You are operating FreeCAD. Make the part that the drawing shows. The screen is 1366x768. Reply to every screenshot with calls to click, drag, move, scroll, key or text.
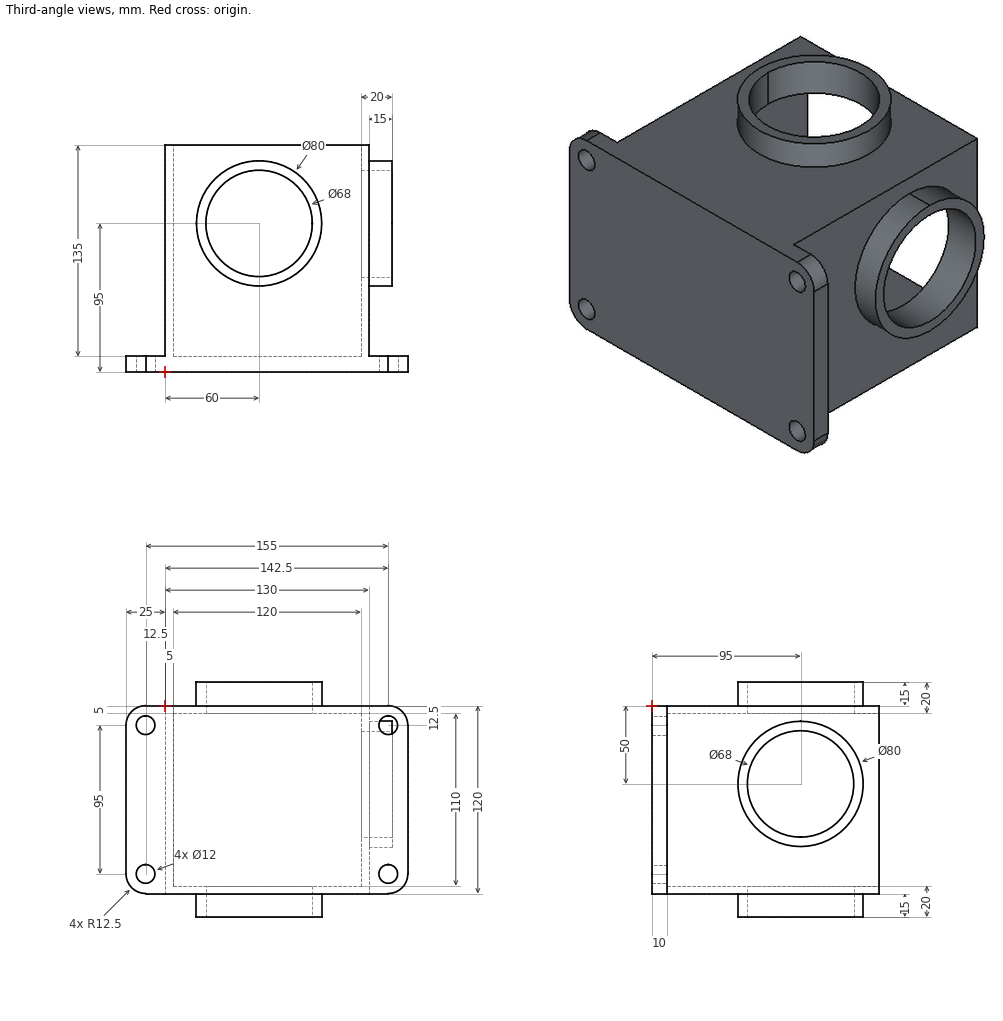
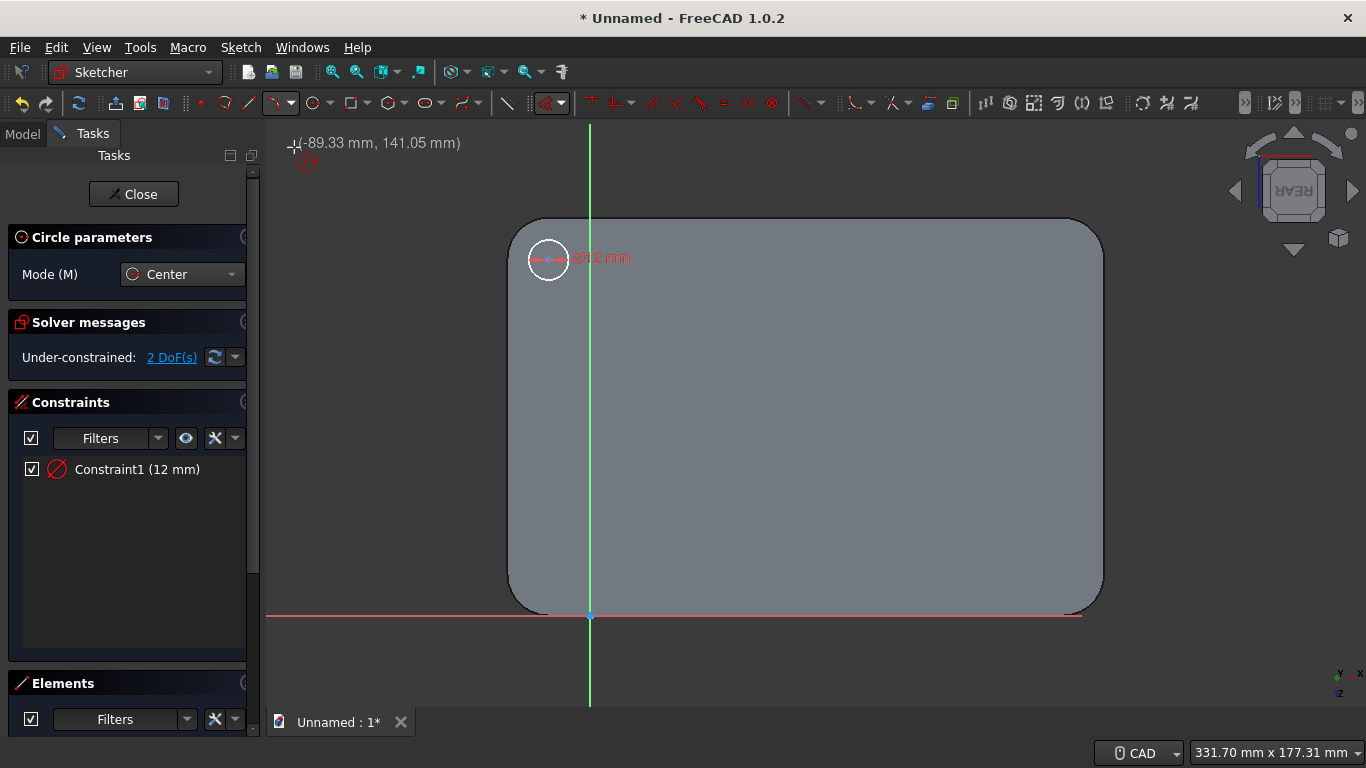
click(1063, 259)
move(1077, 245)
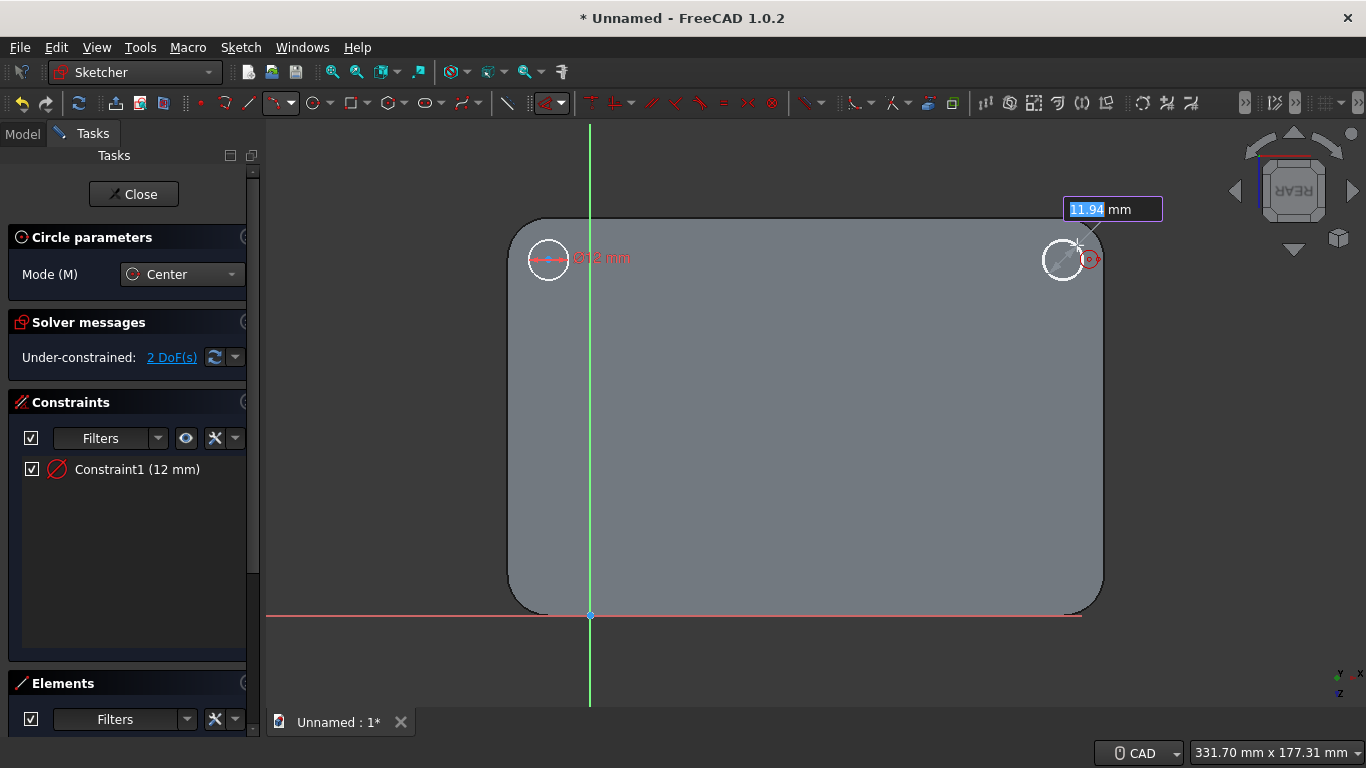
text(12)
key(Return)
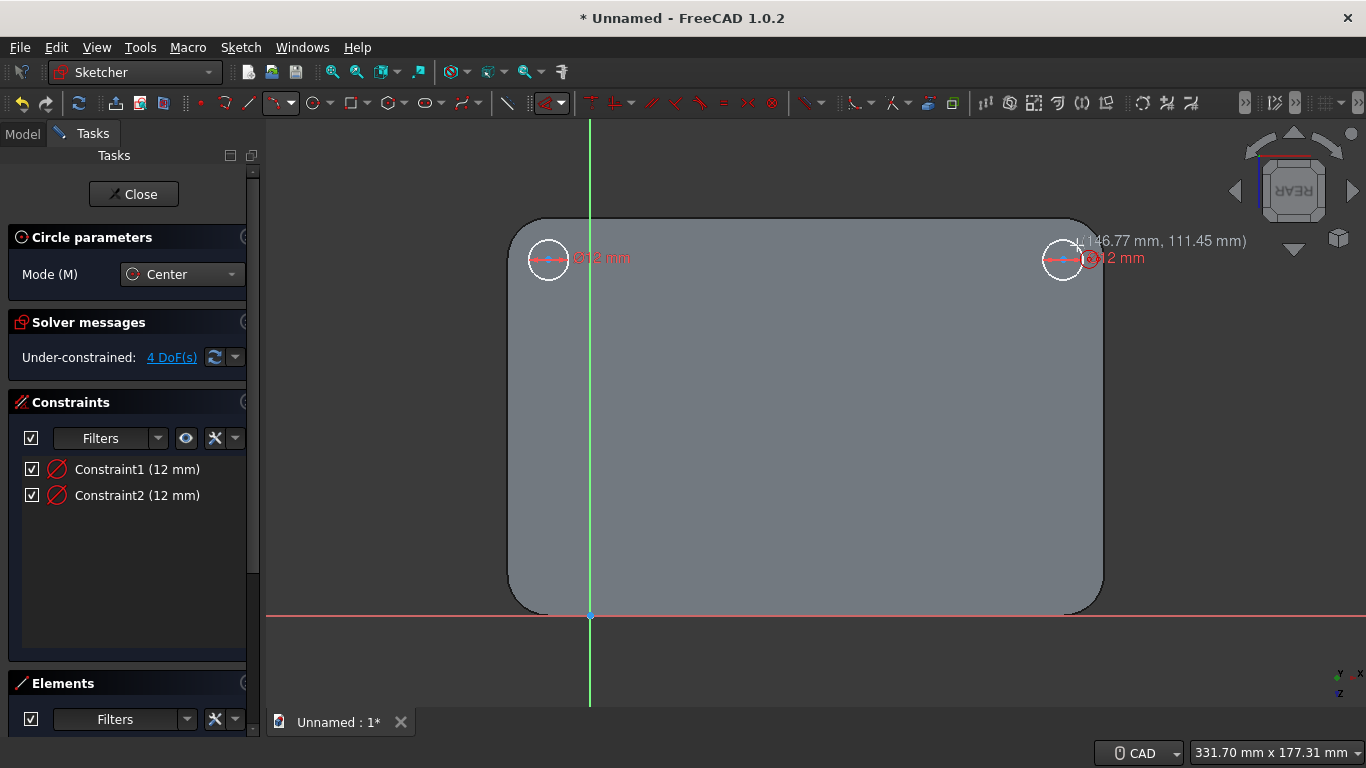
click(1063, 574)
move(1077, 560)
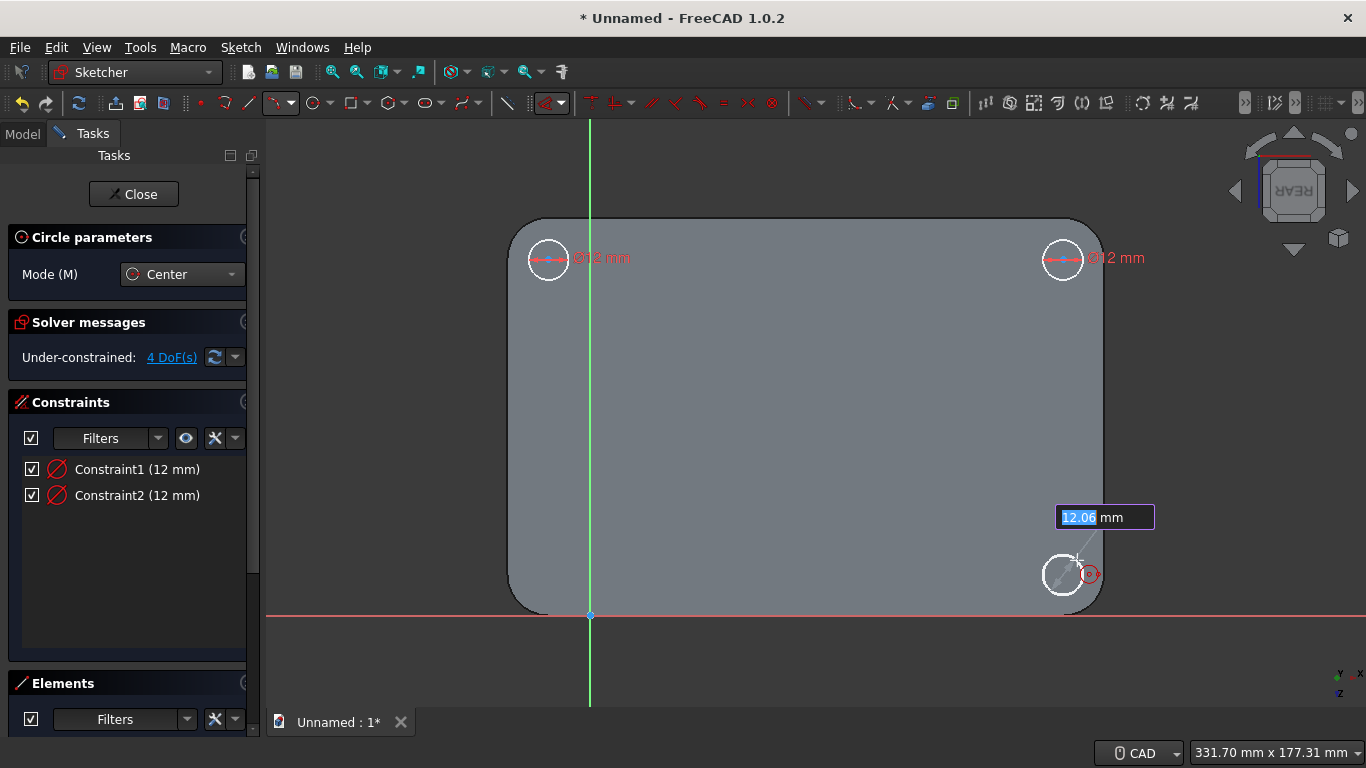
text(12)
key(Return)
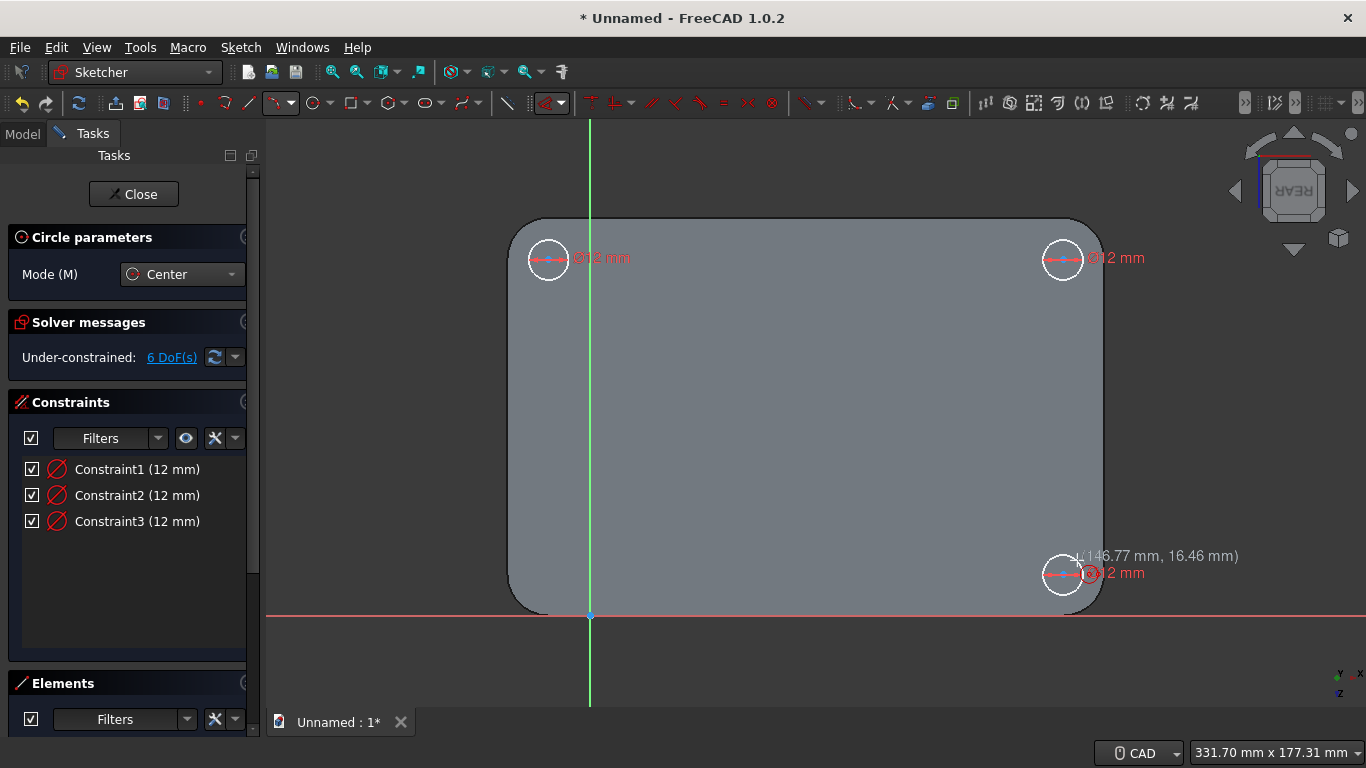
click(549, 574)
move(563, 560)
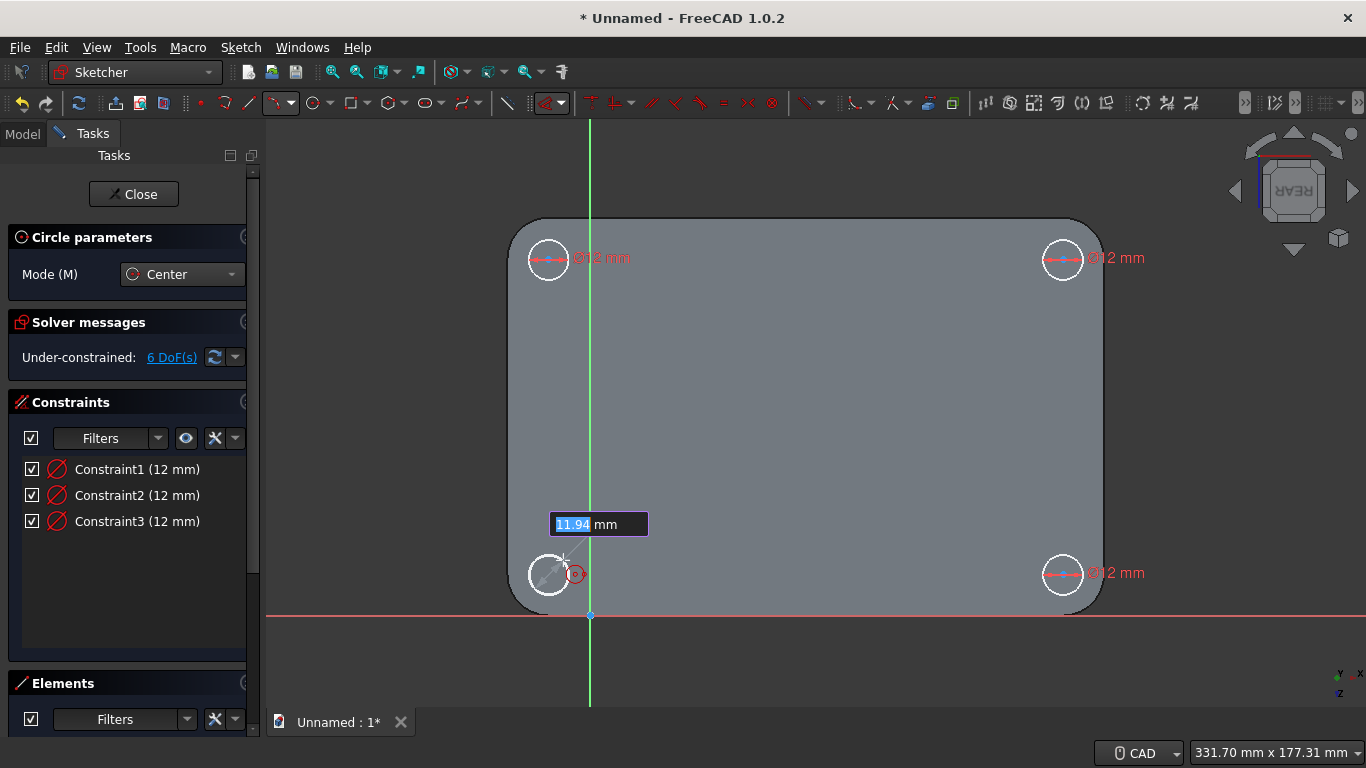
text(12)
key(Return)
key(Escape)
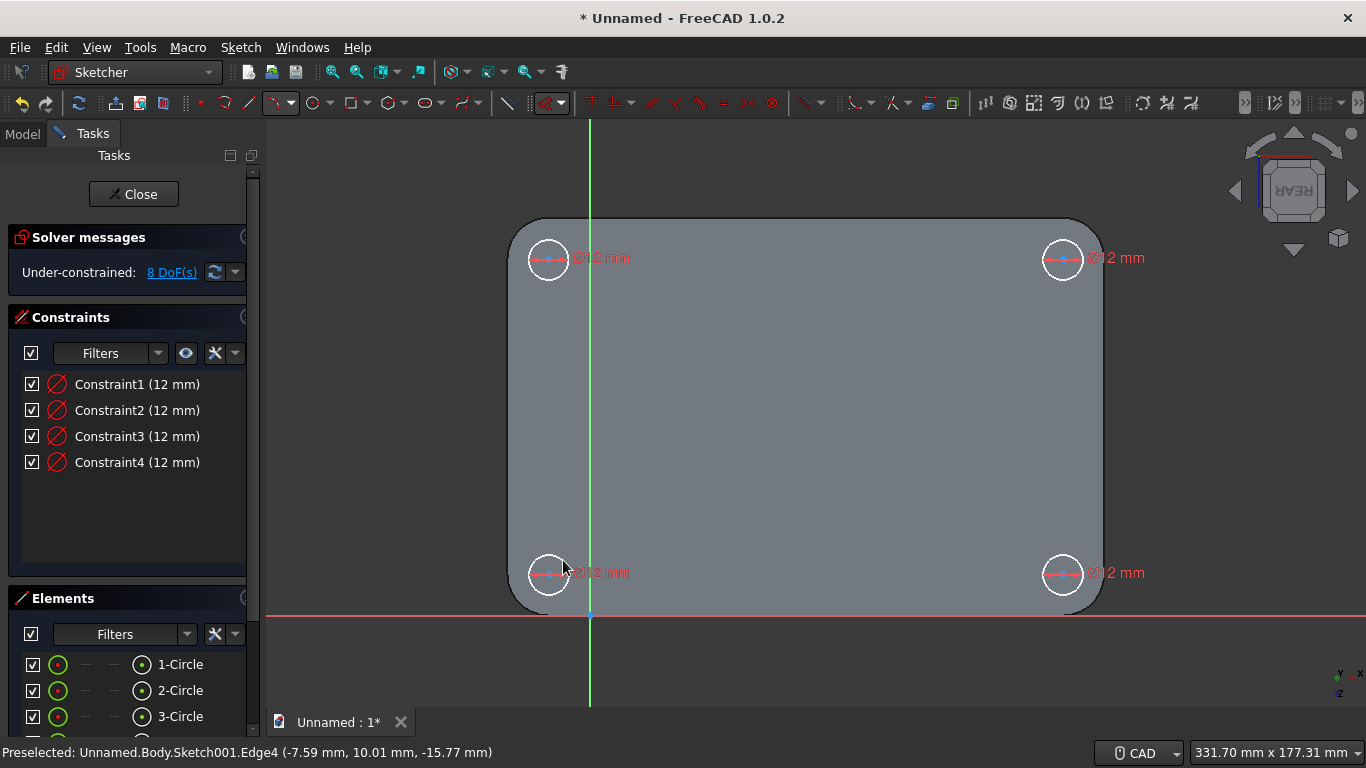
click(1063, 260)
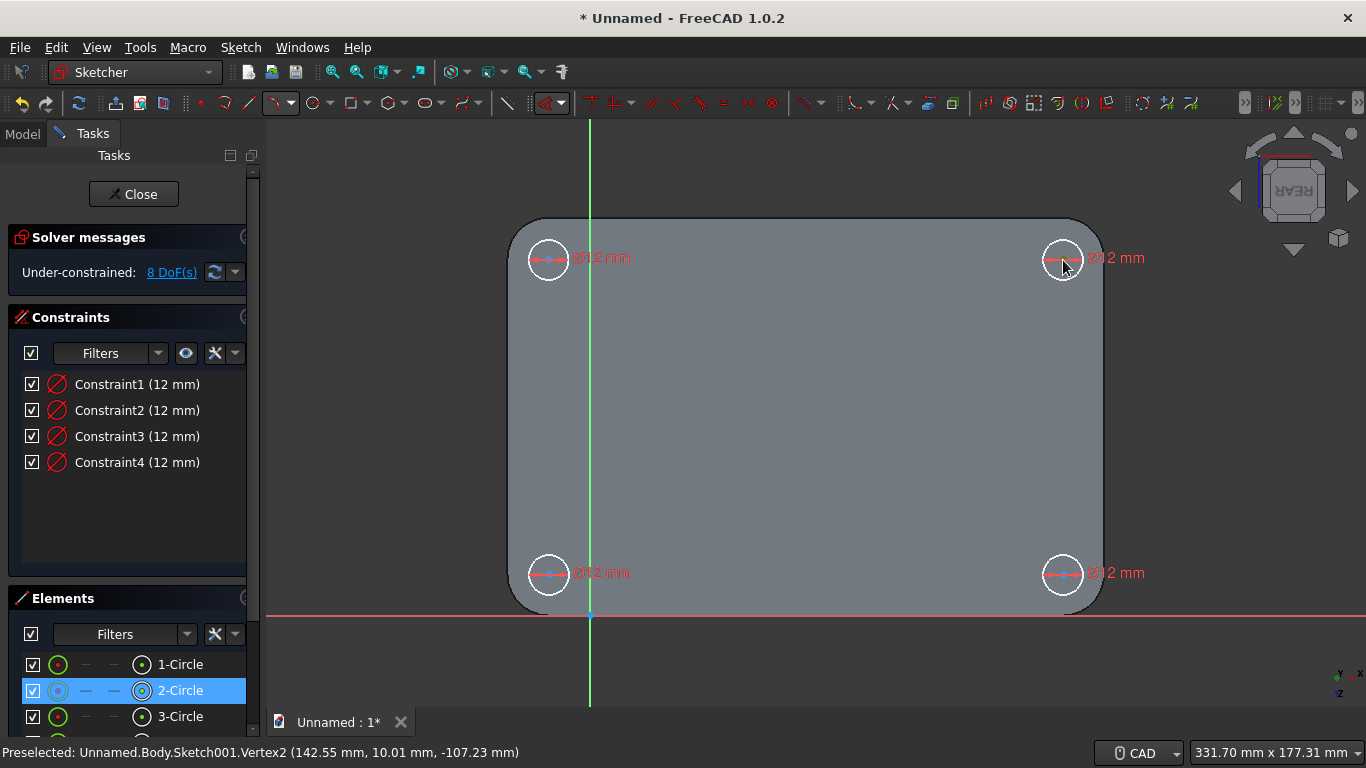
click(1063, 575)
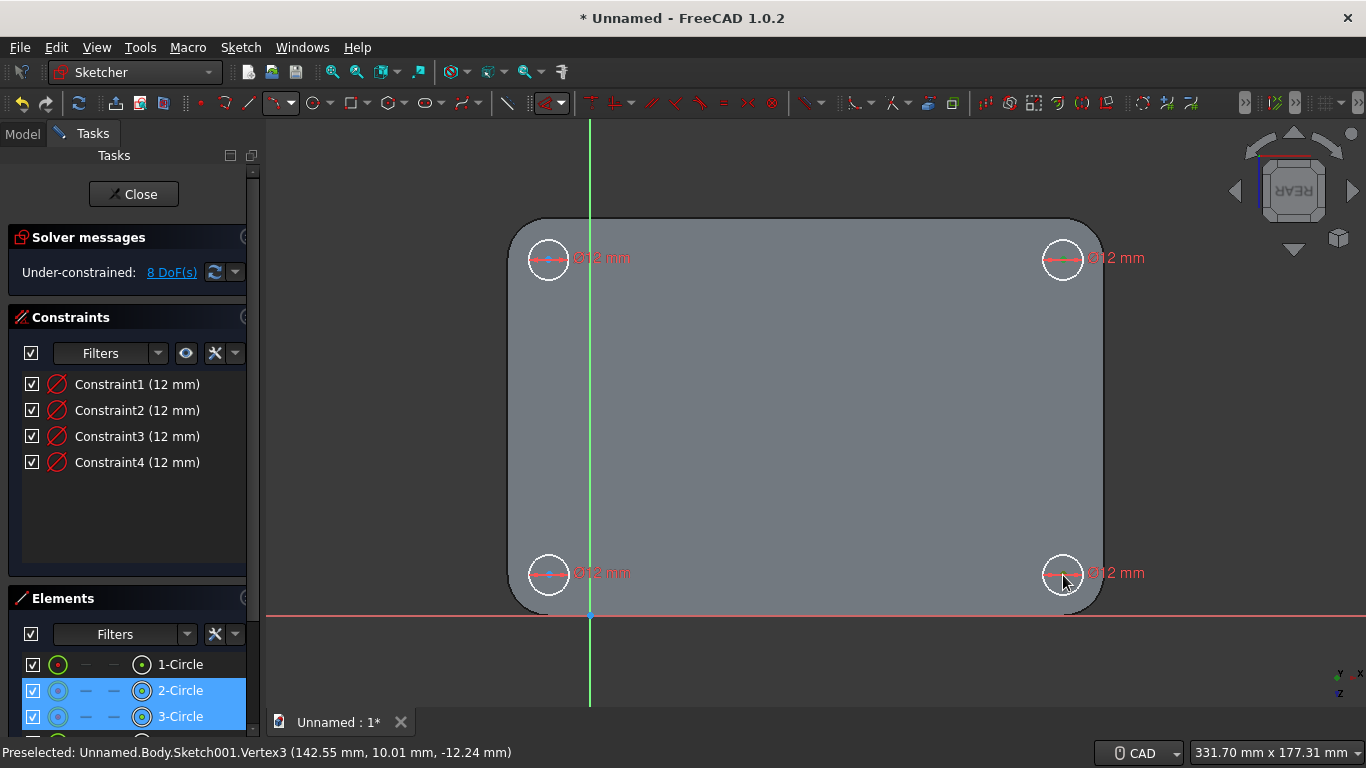
key(i)